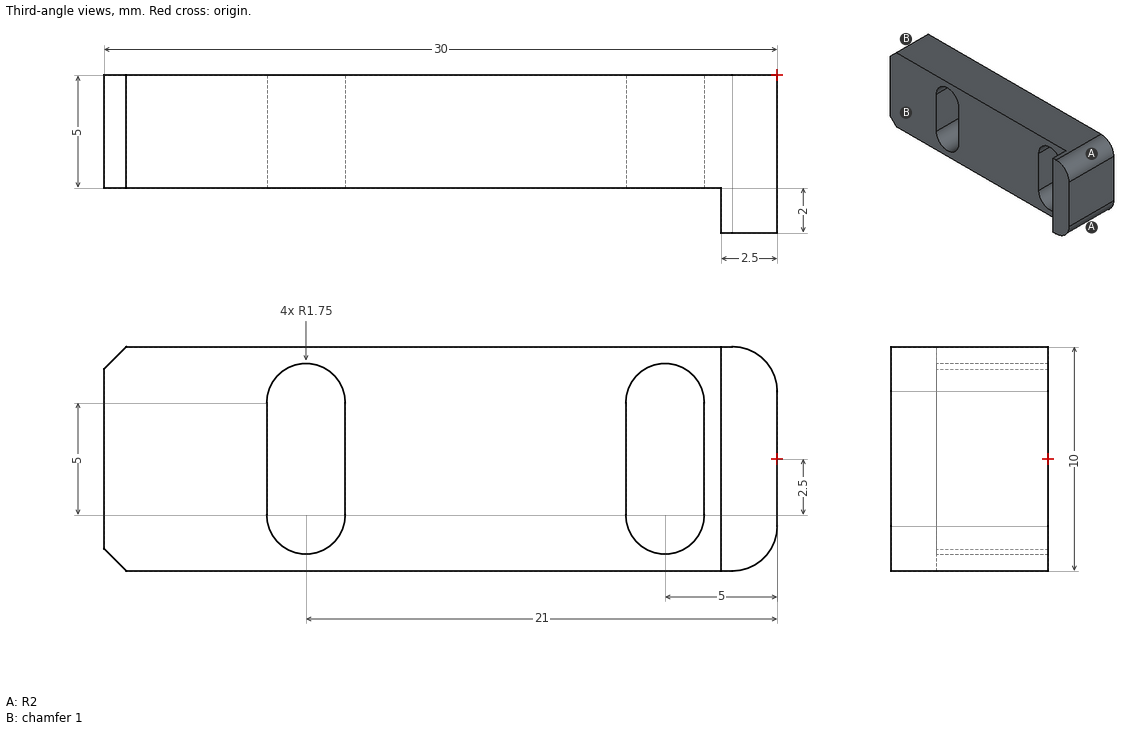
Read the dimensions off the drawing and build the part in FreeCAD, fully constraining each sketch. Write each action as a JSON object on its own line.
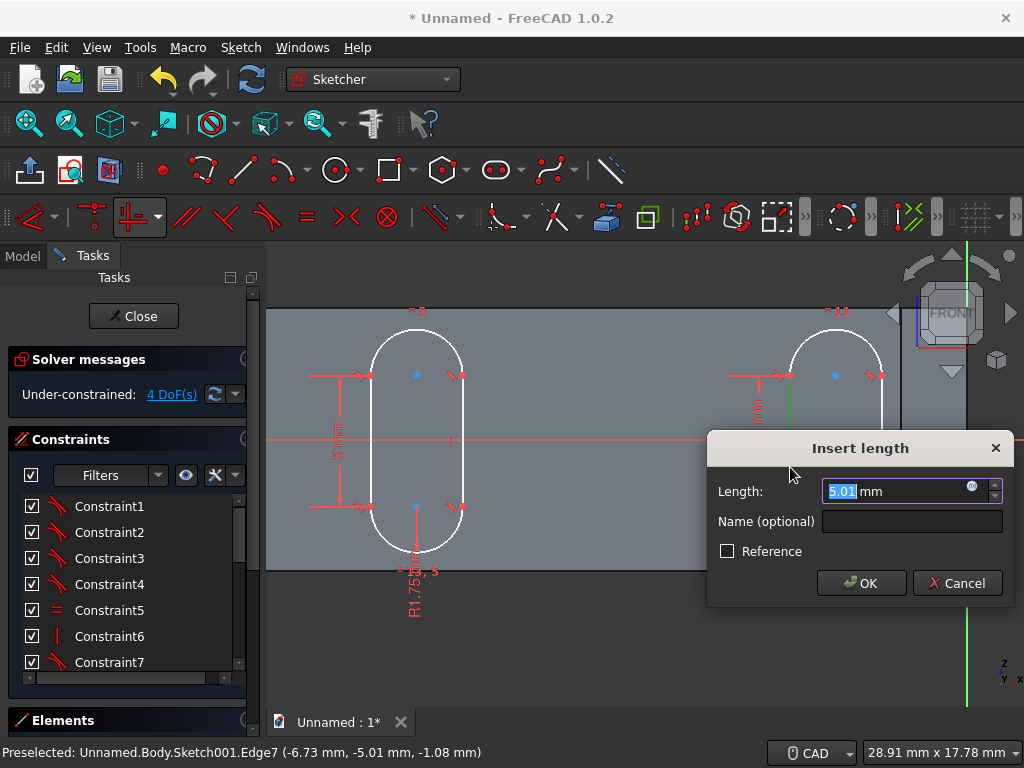
{"action": "type", "text": "5"}
{"action": "key", "text": "Return"}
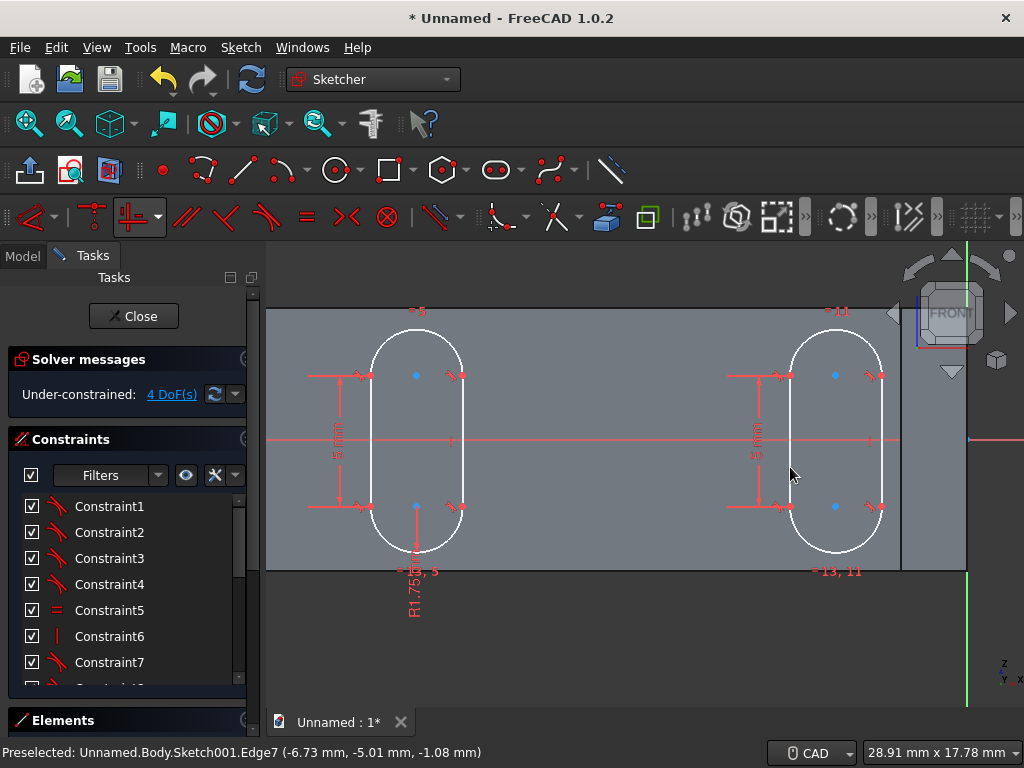
{"action": "left_click", "coordinate": [836, 507]}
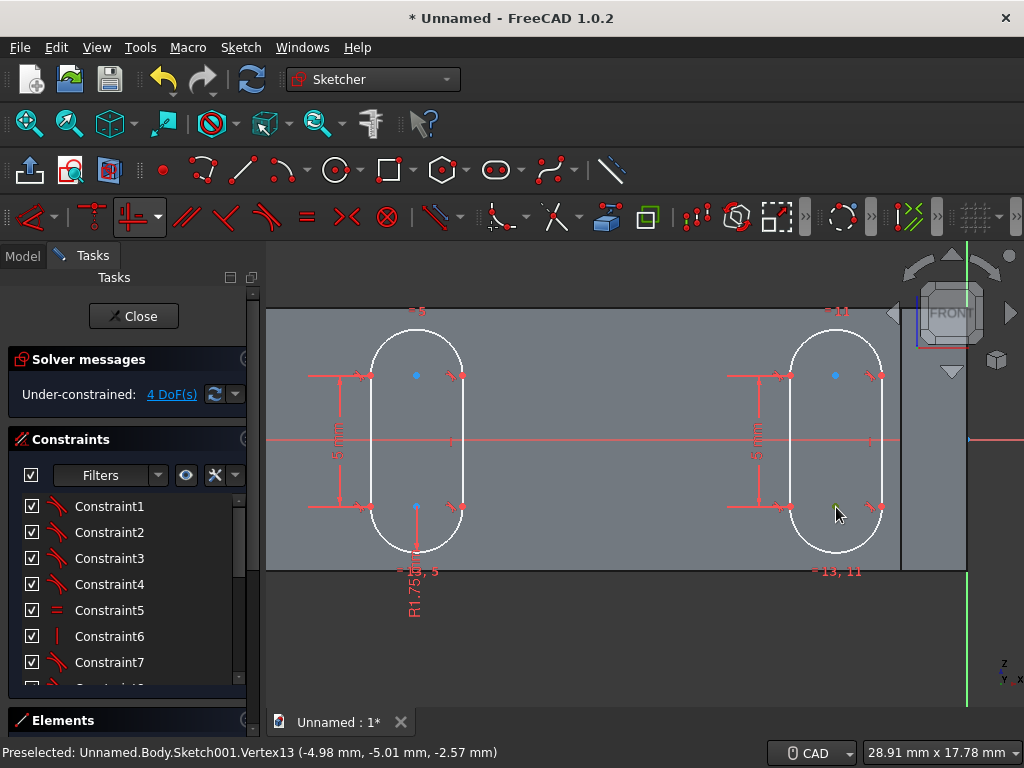
{"action": "left_click", "coordinate": [56, 218]}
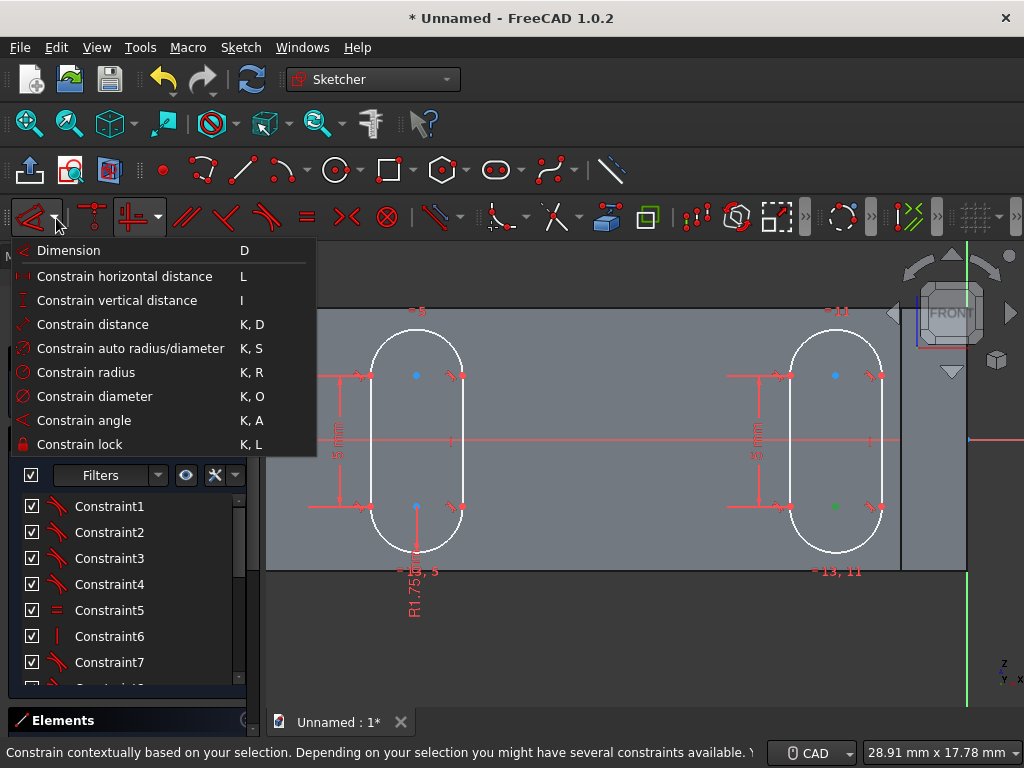
{"action": "left_click", "coordinate": [164, 276]}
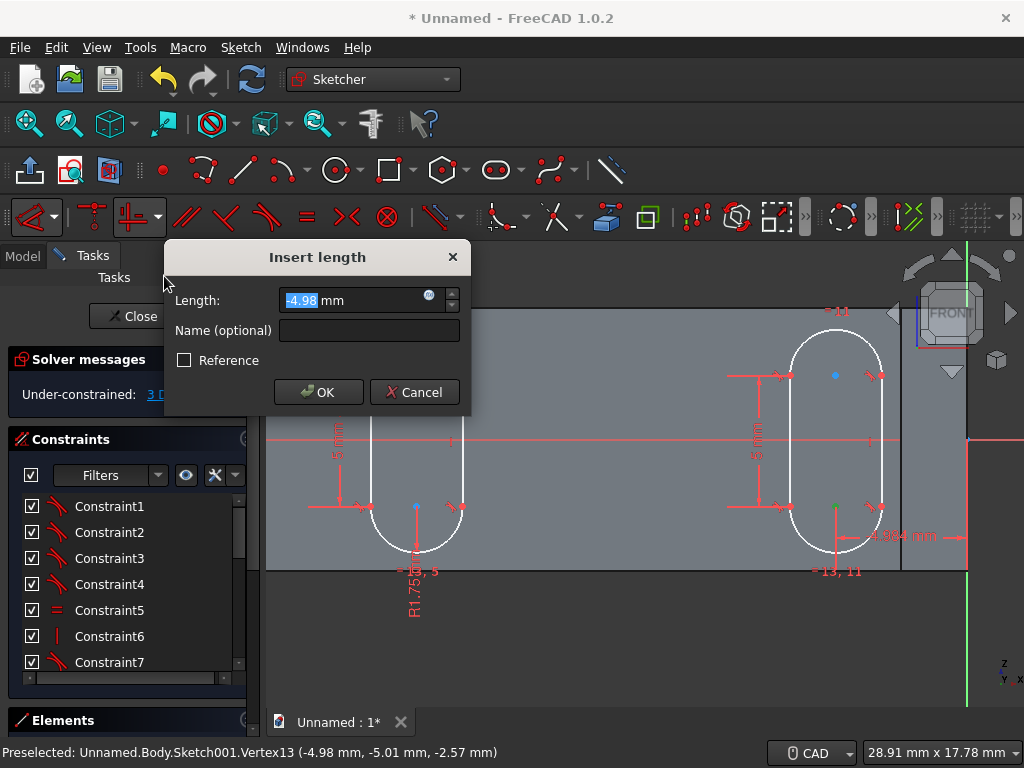
{"action": "type", "text": "-5"}
{"action": "key", "text": "Return"}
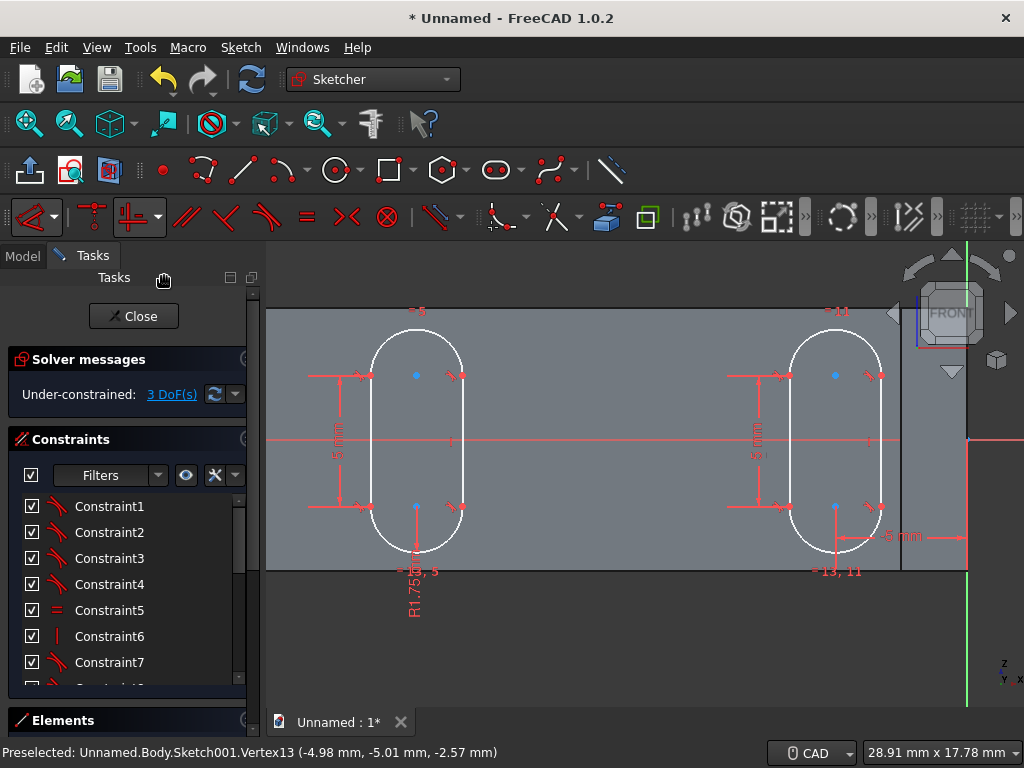
{"action": "left_click", "coordinate": [417, 507]}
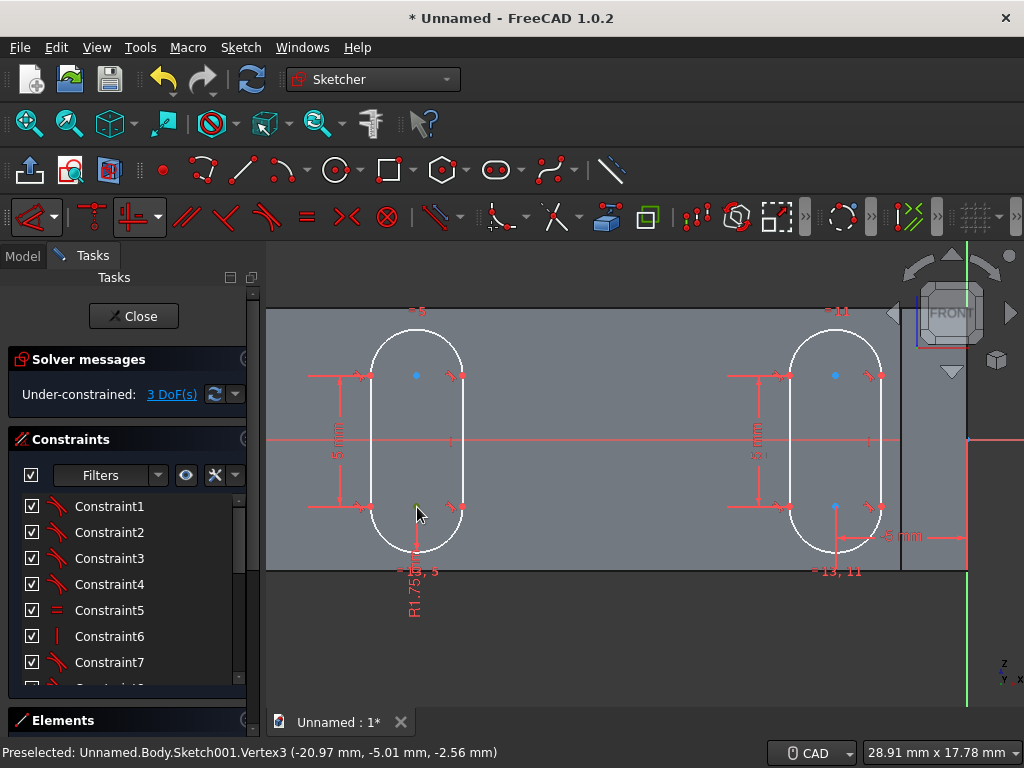
{"action": "key", "text": "l"}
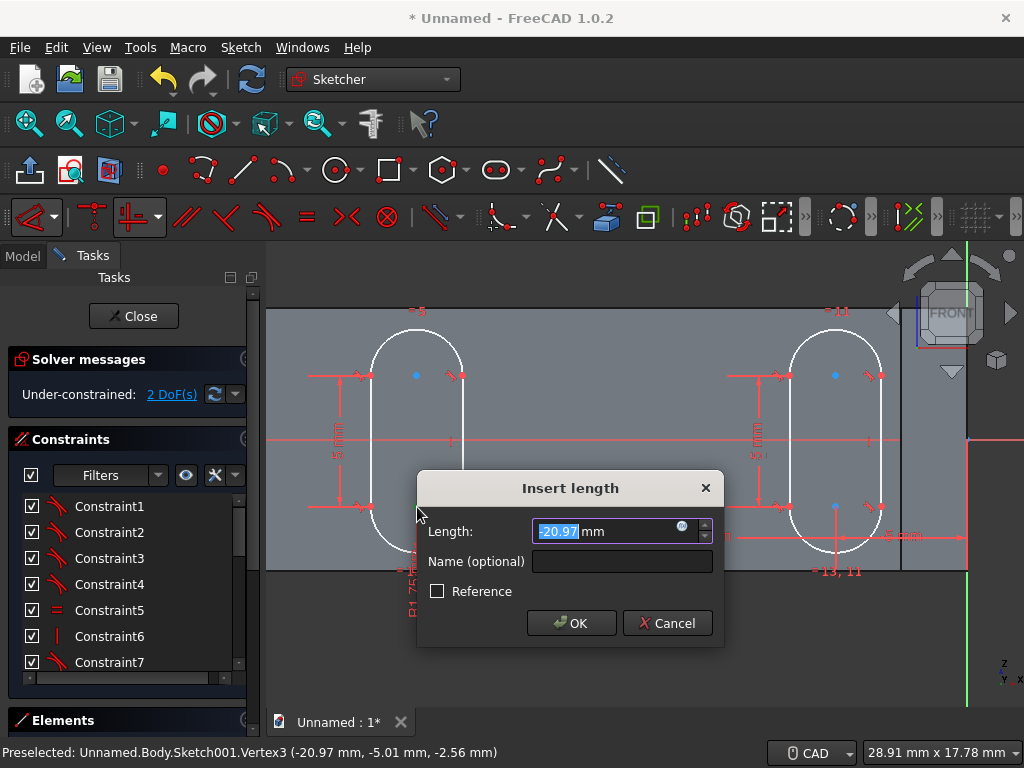
{"action": "type", "text": "-21"}
{"action": "key", "text": "Return"}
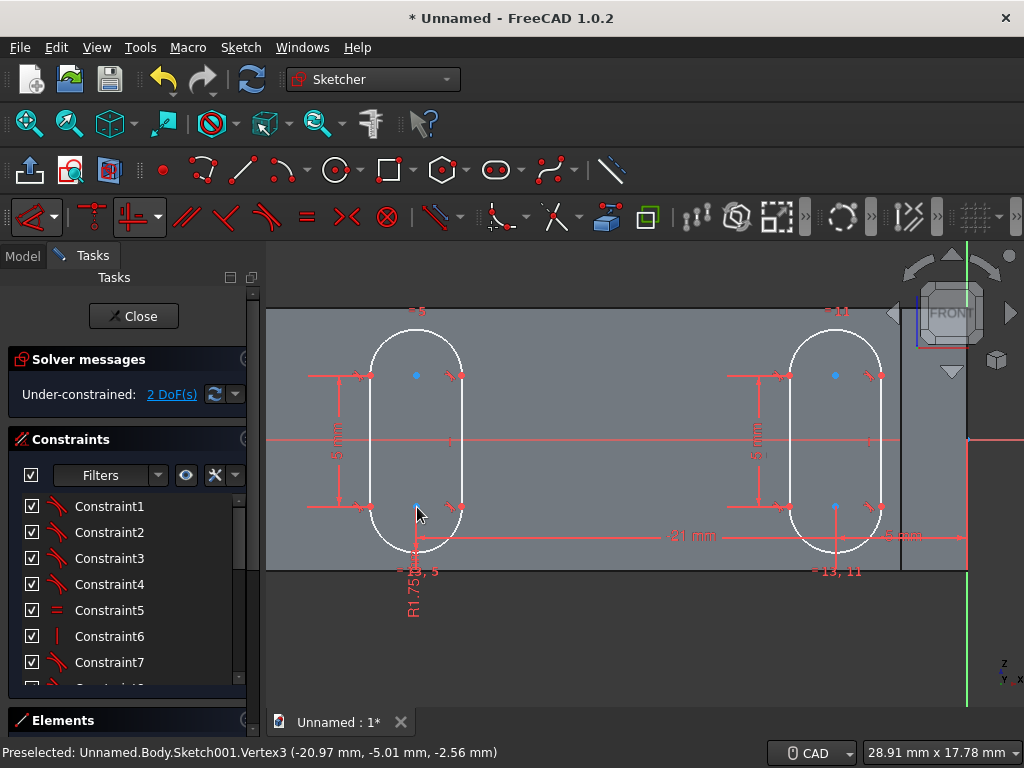
{"action": "left_click", "coordinate": [370, 507]}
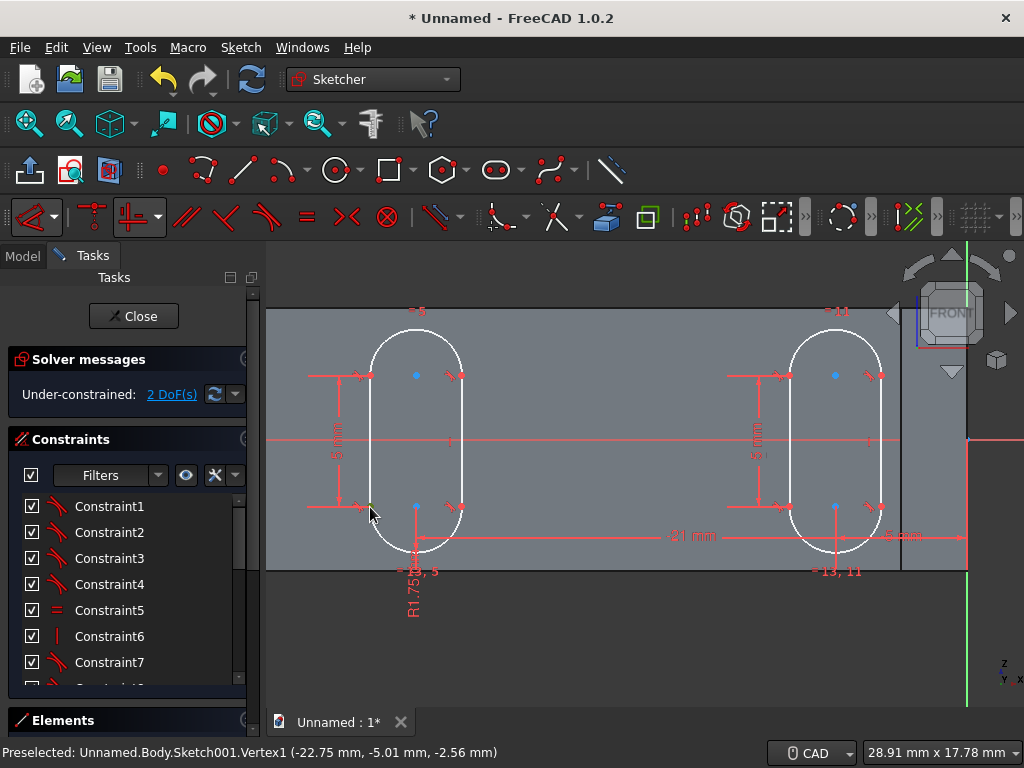
{"action": "key", "text": "i"}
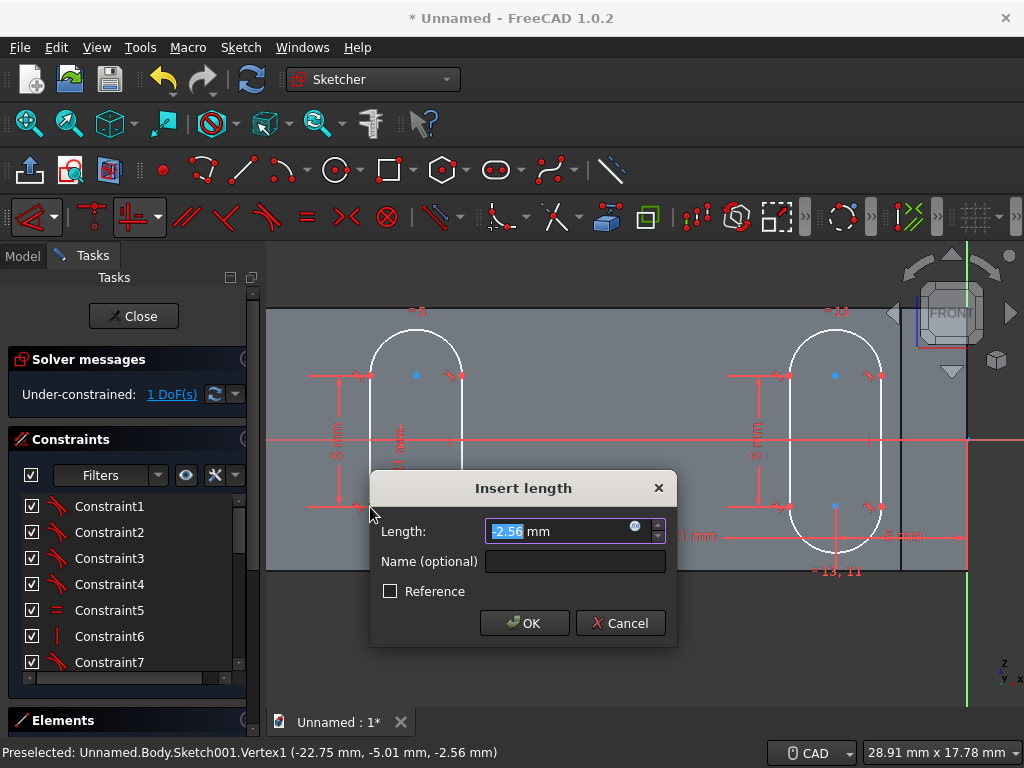
{"action": "type", "text": "-2.5"}
{"action": "key", "text": "Return"}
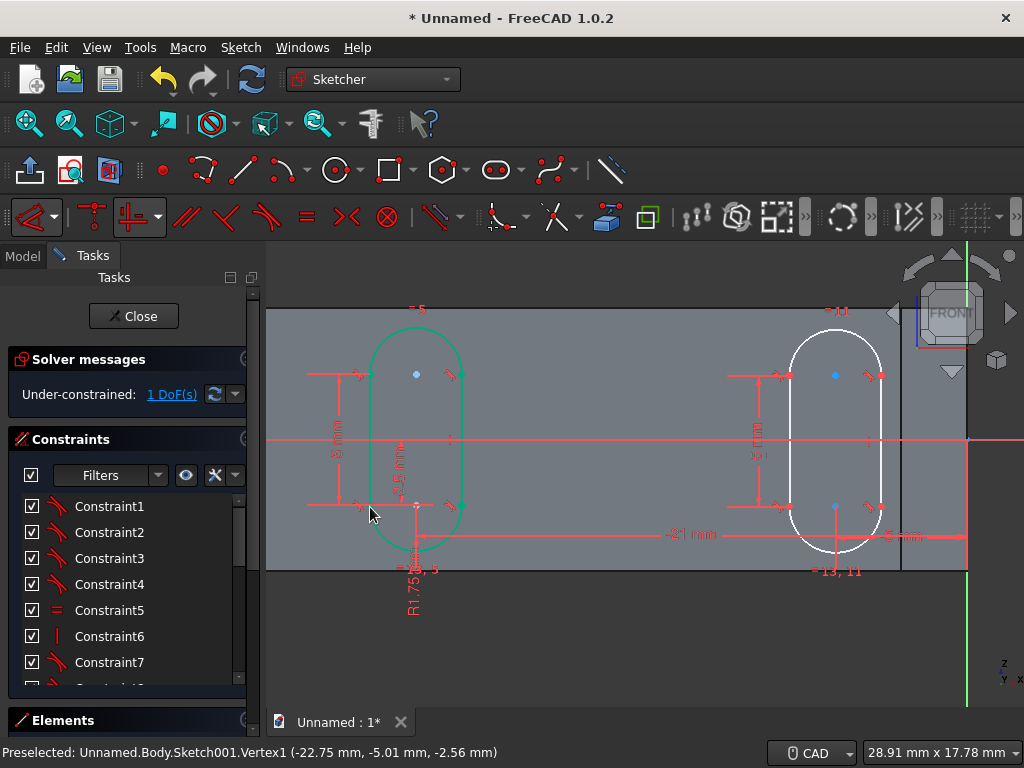
{"action": "left_click", "coordinate": [790, 507]}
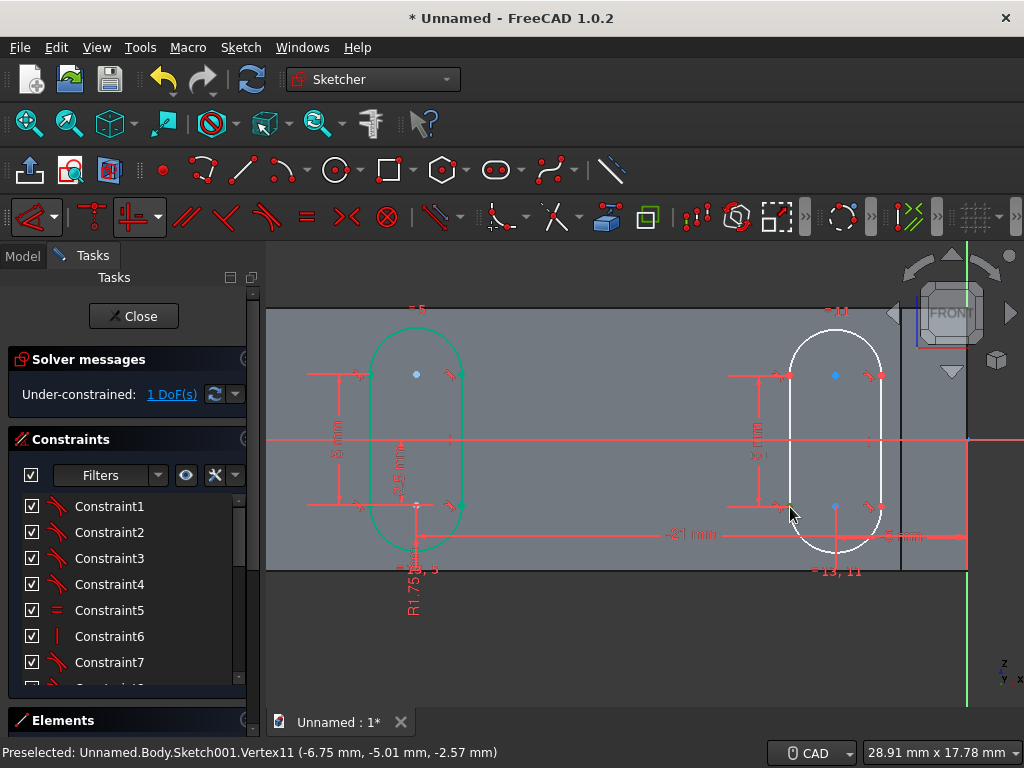
{"action": "key", "text": "i"}